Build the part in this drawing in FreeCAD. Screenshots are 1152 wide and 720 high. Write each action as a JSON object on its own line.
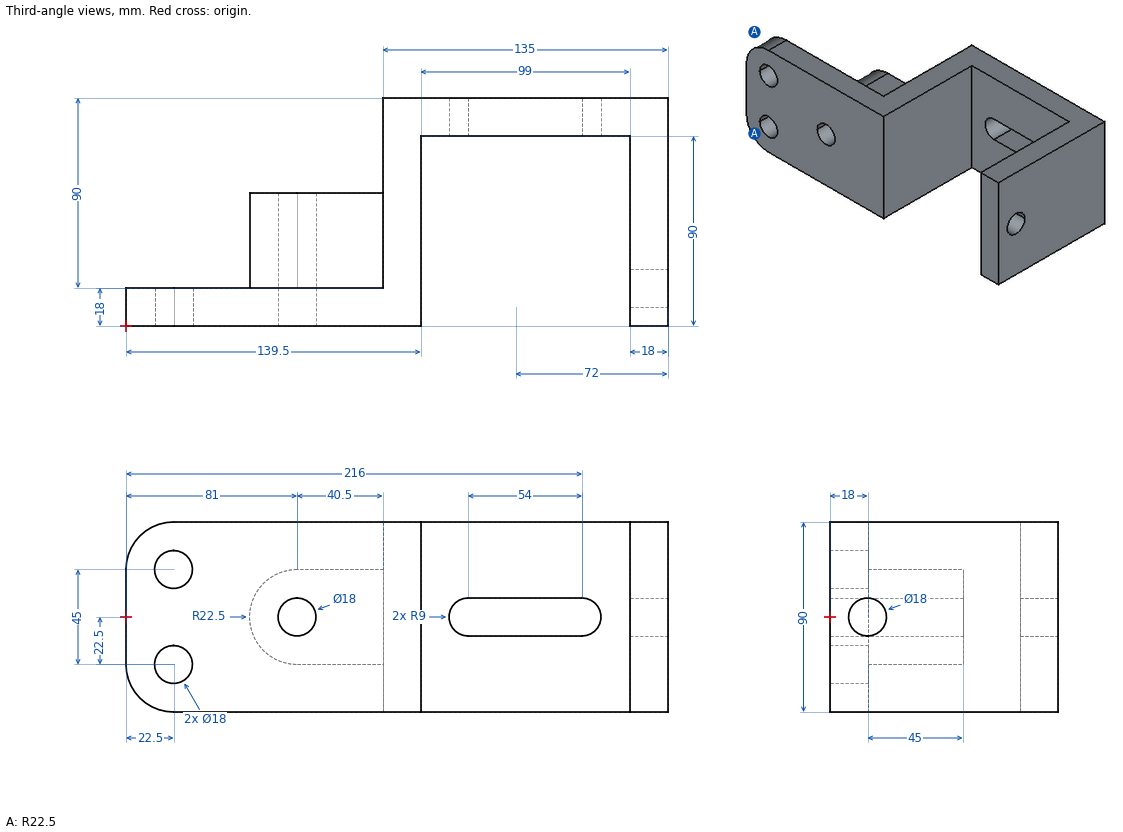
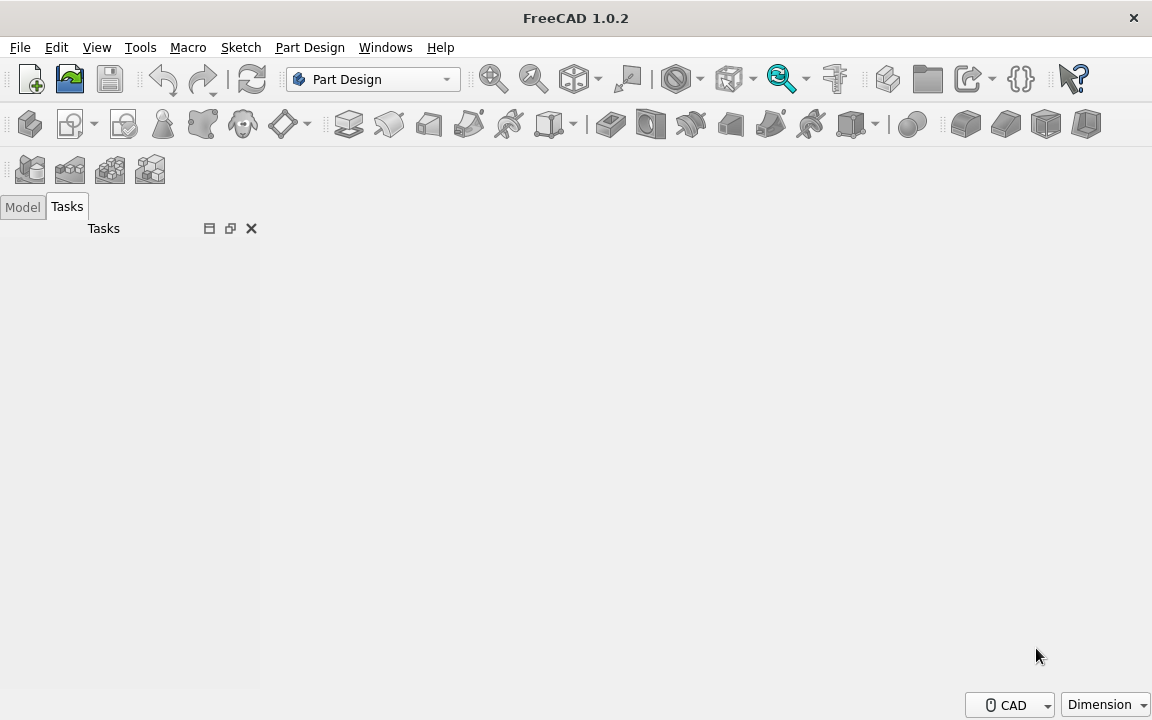
{"action": "left_click", "coordinate": [30, 80]}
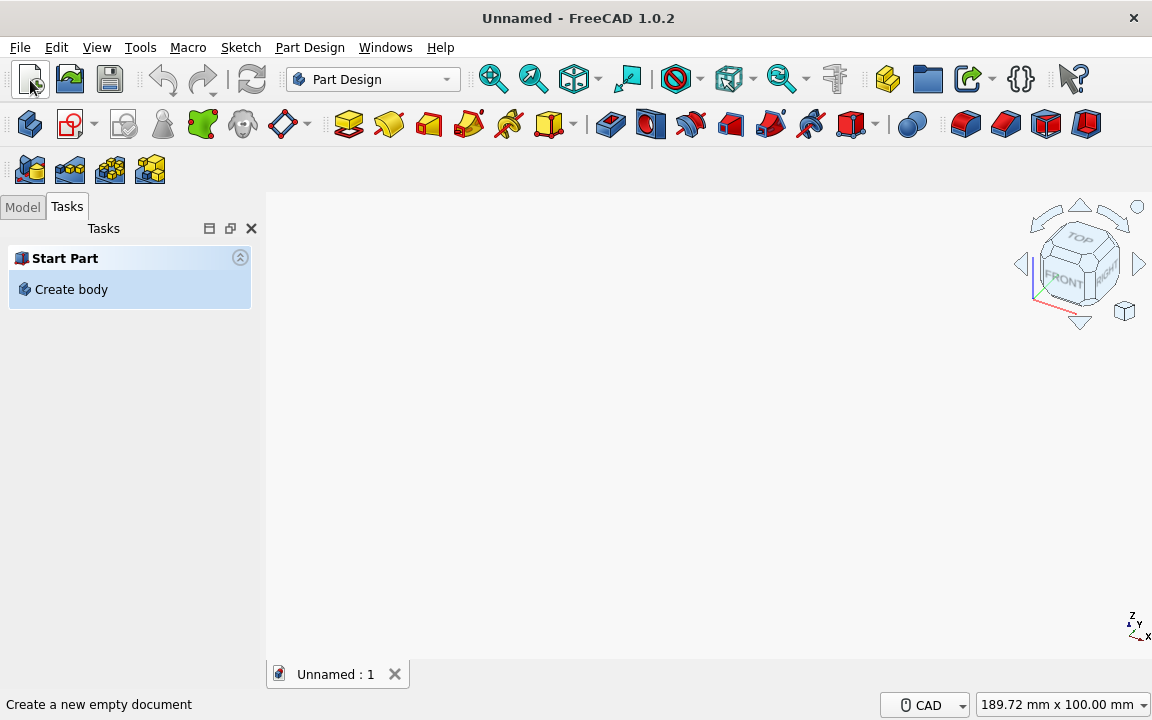
{"action": "left_click", "coordinate": [70, 124]}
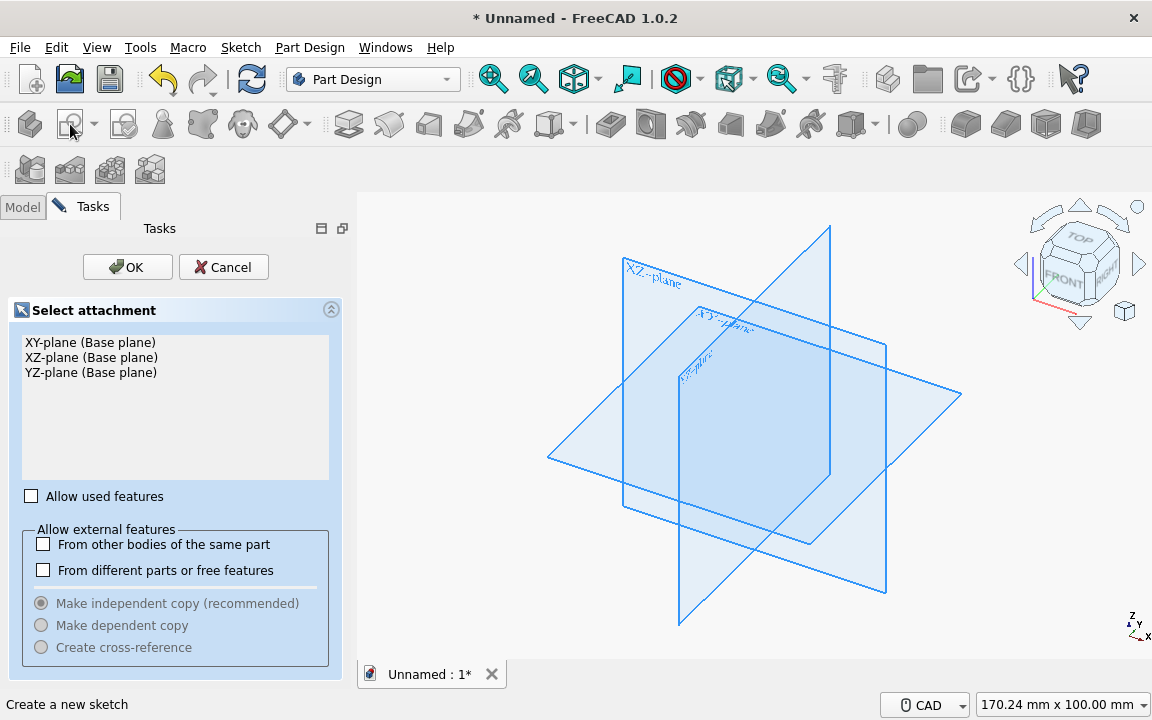
{"action": "left_click", "coordinate": [82, 342]}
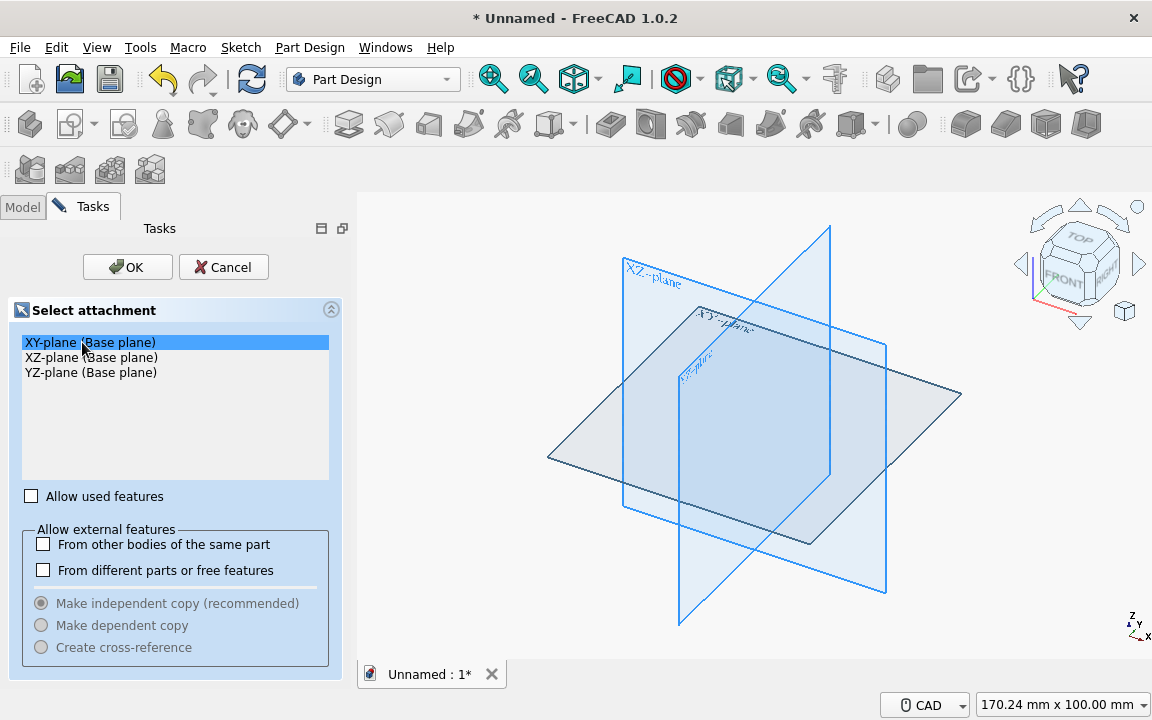
{"action": "left_click", "coordinate": [128, 267]}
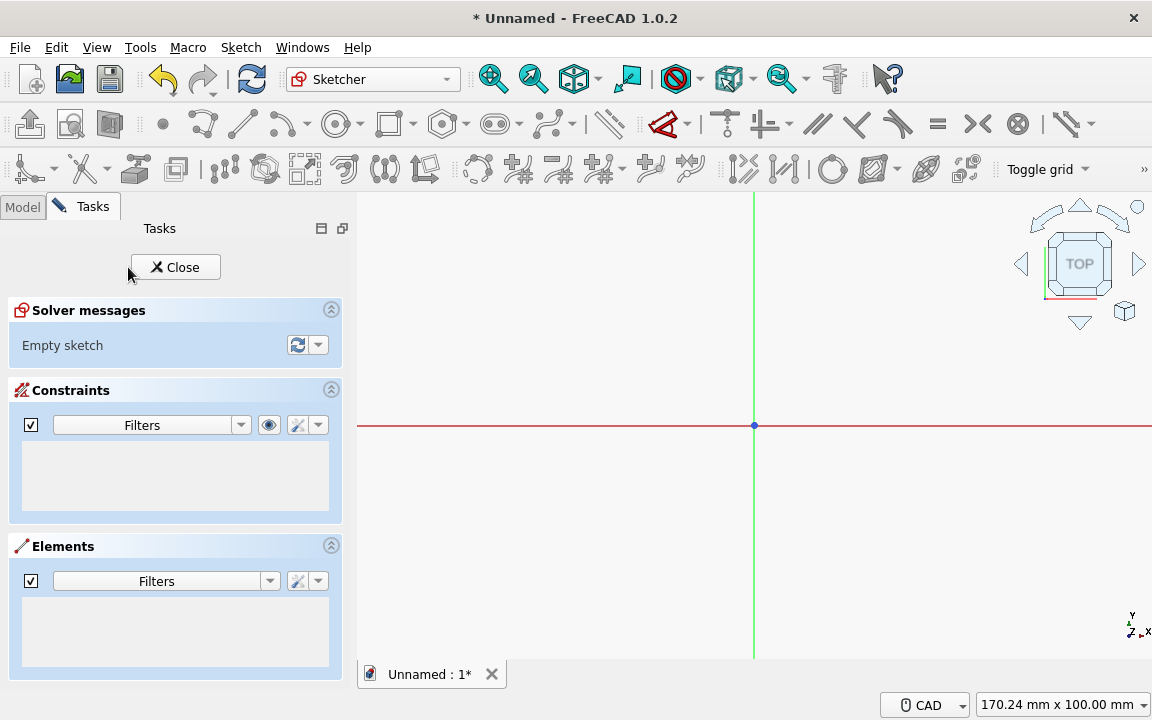
{"action": "scroll", "coordinate": [294, 572], "scroll_direction": "down", "scroll_amount": 5}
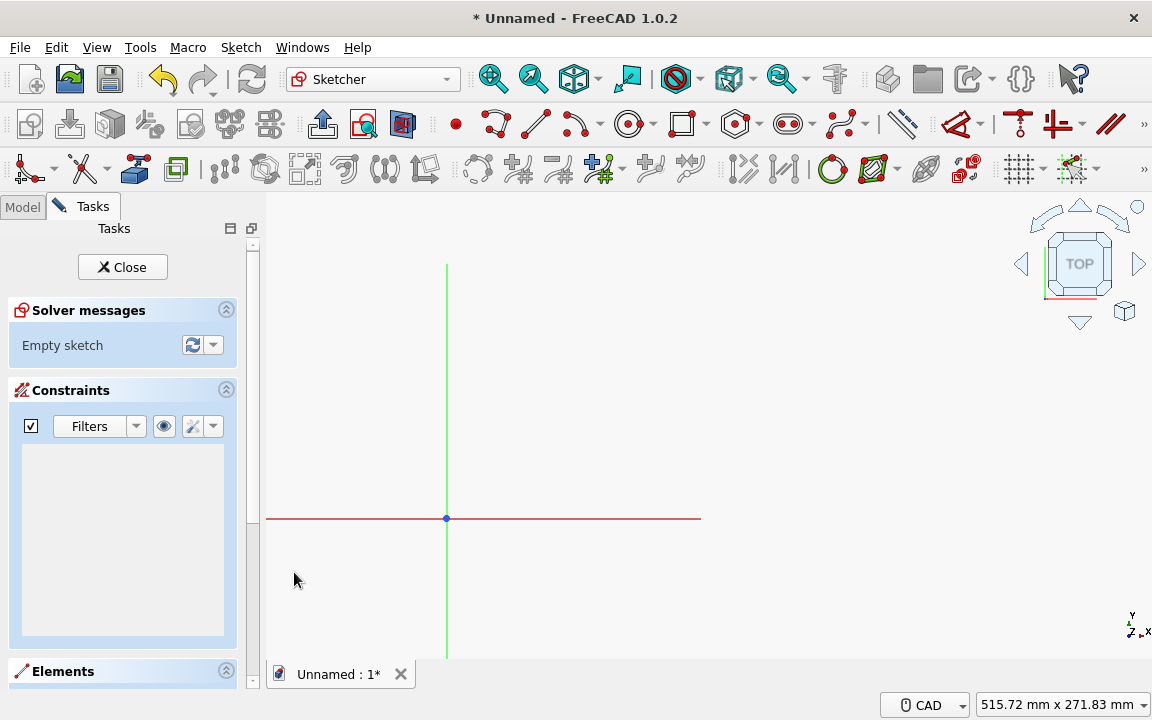
{"action": "key", "text": "g m"}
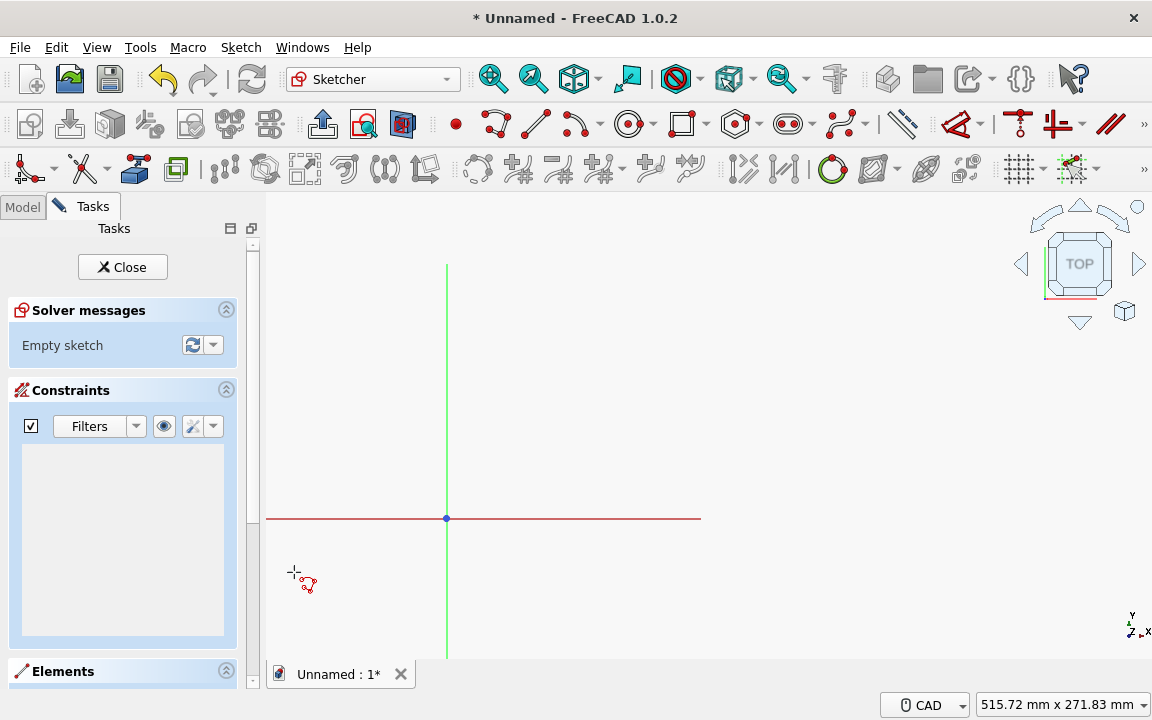
{"action": "left_click", "coordinate": [447, 519]}
{"action": "left_click", "coordinate": [686, 510]}
{"action": "left_click", "coordinate": [686, 364]}
{"action": "left_click", "coordinate": [856, 364]}
{"action": "left_click", "coordinate": [856, 519]}
{"action": "left_click", "coordinate": [887, 510]}
{"action": "left_click", "coordinate": [887, 333]}
{"action": "left_click", "coordinate": [655, 333]}
{"action": "left_click", "coordinate": [655, 488]}
{"action": "left_click", "coordinate": [456, 488]}
{"action": "left_click", "coordinate": [447, 519]}
{"action": "key", "text": "Escape"}
{"action": "key", "text": "Escape"}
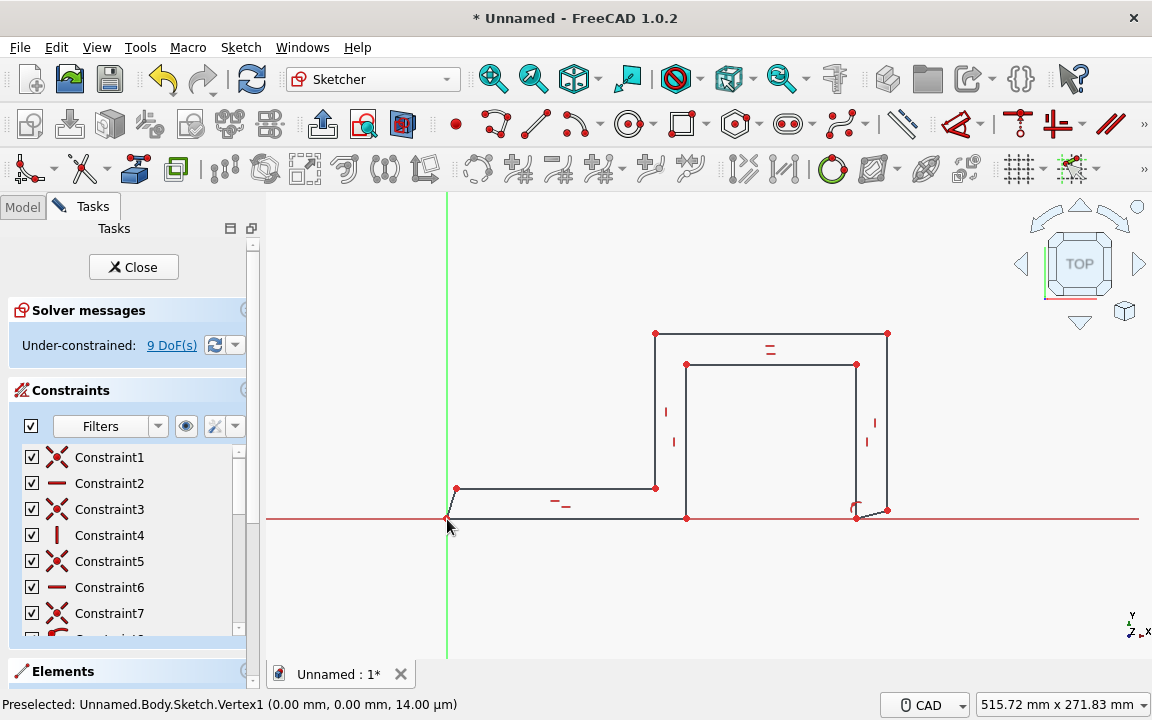
{"action": "scroll", "coordinate": [865, 516], "scroll_direction": "up", "scroll_amount": 2}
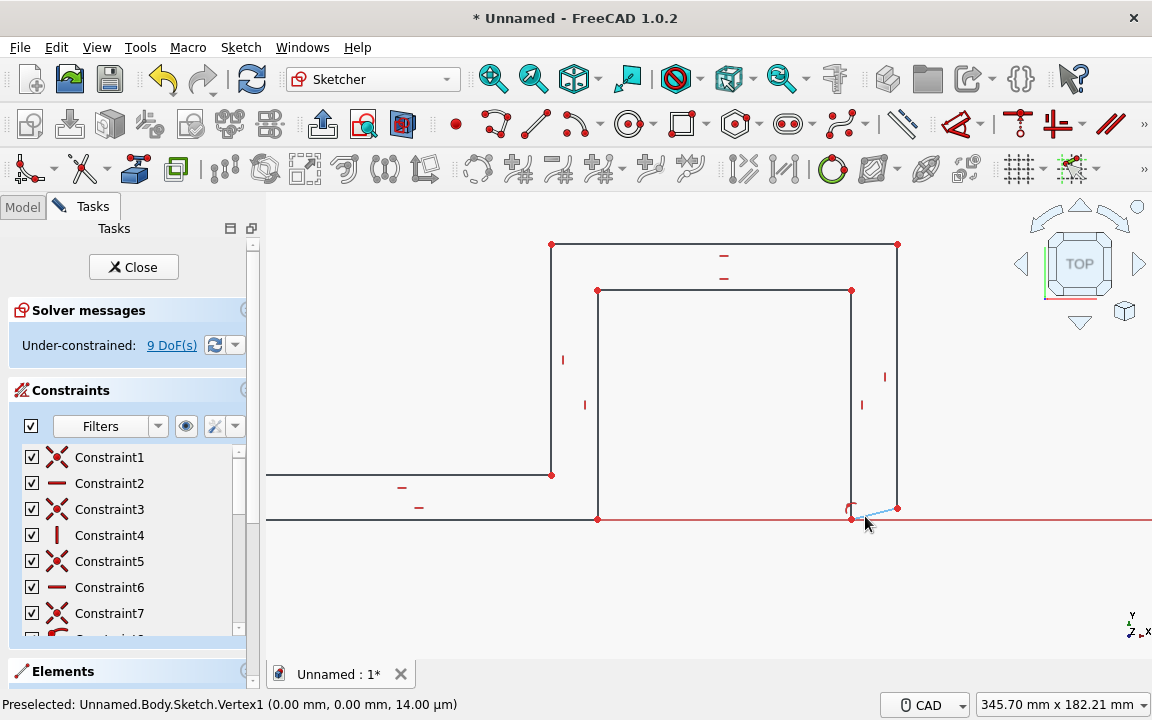
{"action": "left_click", "coordinate": [865, 516]}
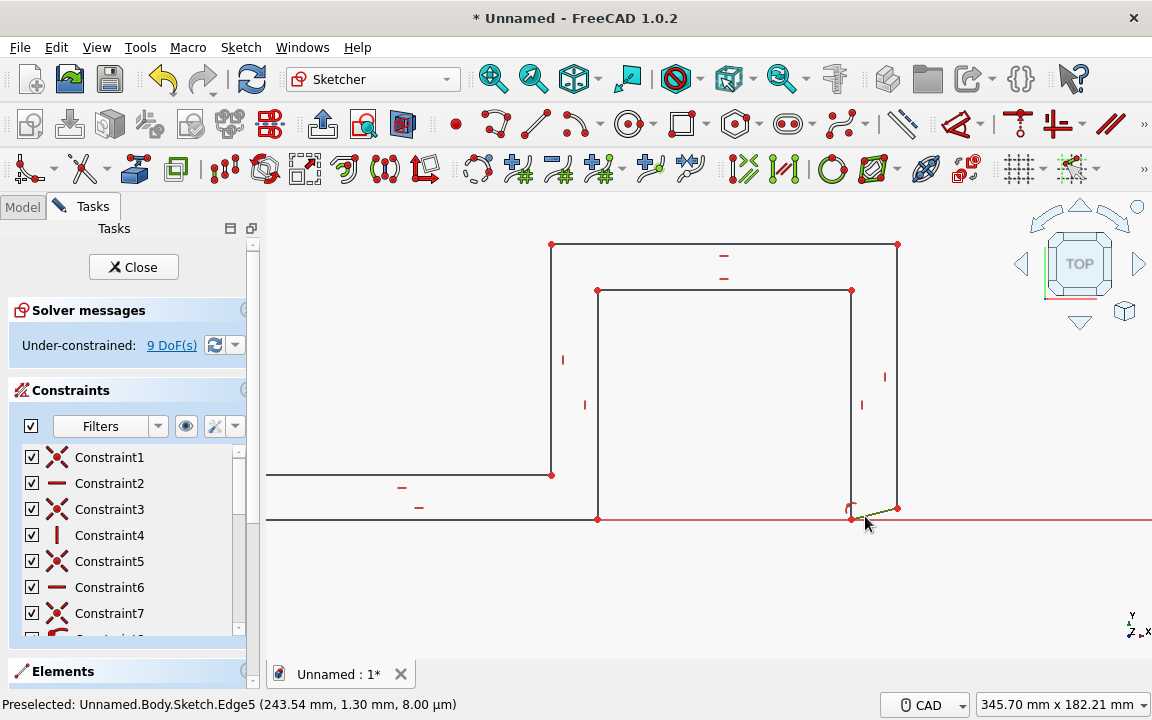
{"action": "left_click", "coordinate": [1084, 124]}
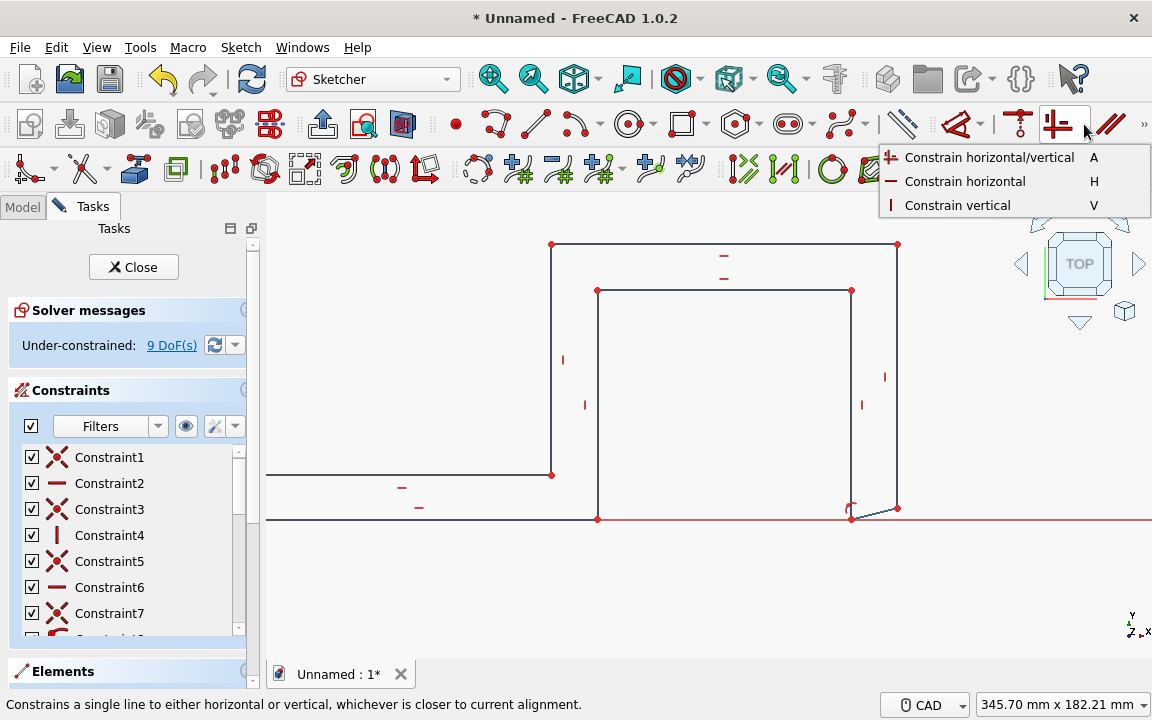
{"action": "left_click", "coordinate": [1015, 181]}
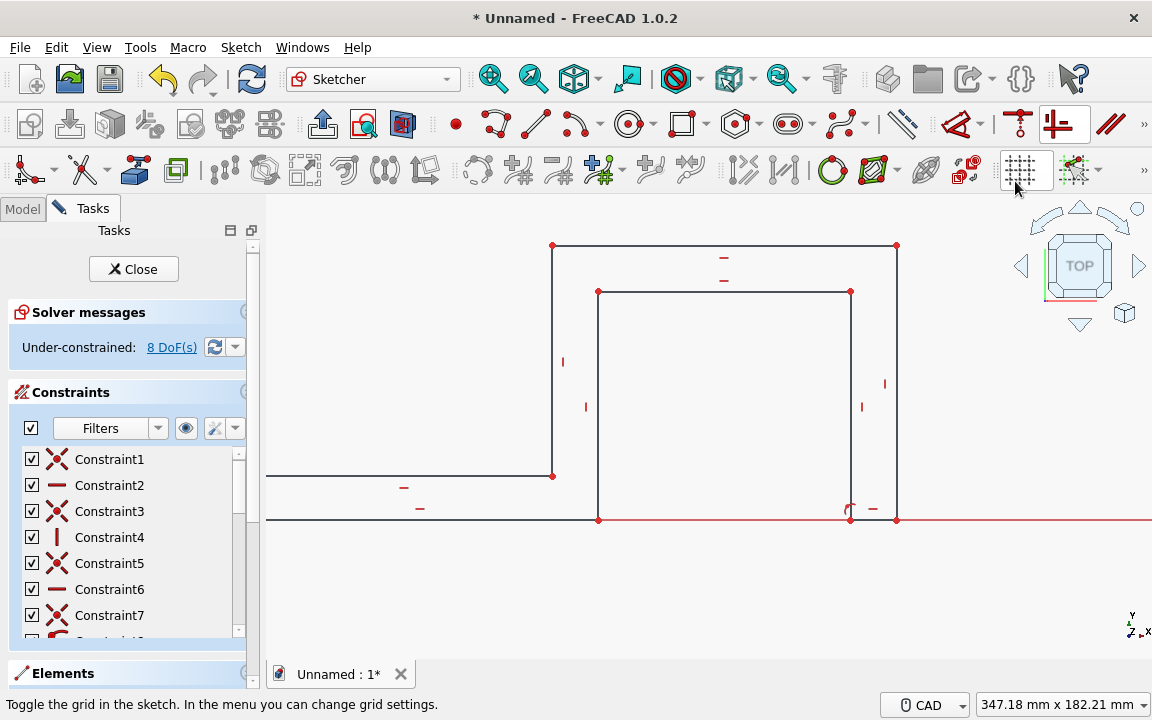
{"action": "scroll", "coordinate": [959, 626], "scroll_direction": "down", "scroll_amount": 1}